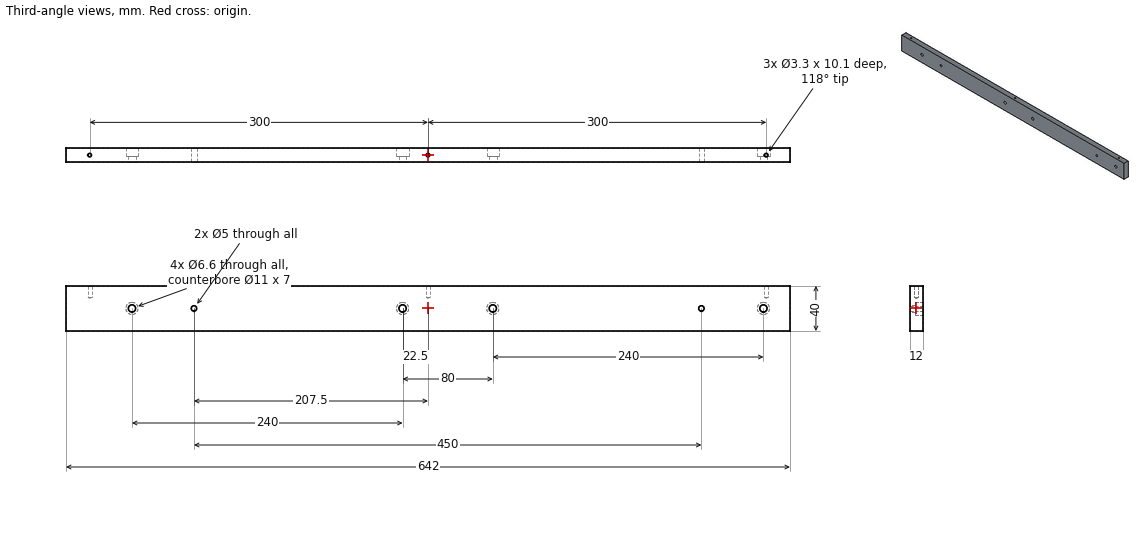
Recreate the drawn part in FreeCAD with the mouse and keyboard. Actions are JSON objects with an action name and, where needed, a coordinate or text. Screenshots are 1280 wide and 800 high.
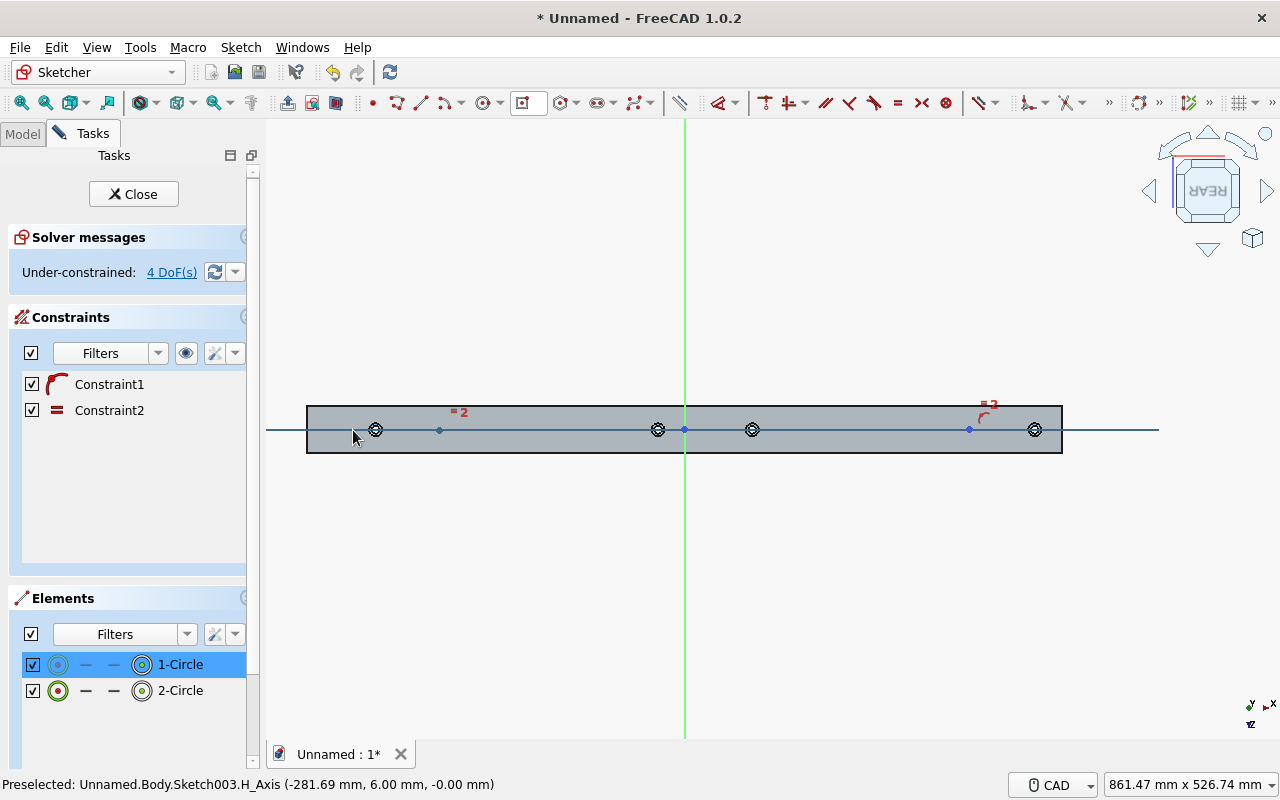
{"action": "left_click", "coordinate": [766, 104]}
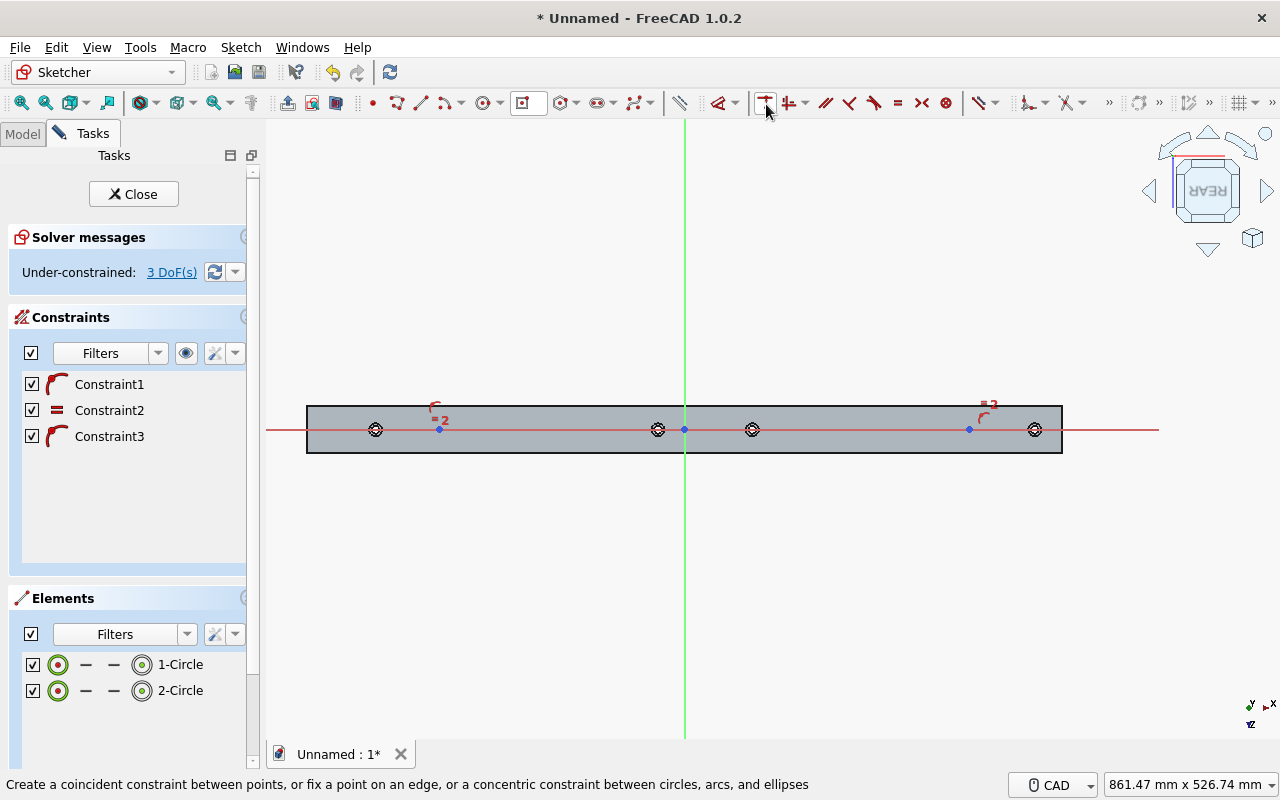
{"action": "left_click", "coordinate": [718, 104]}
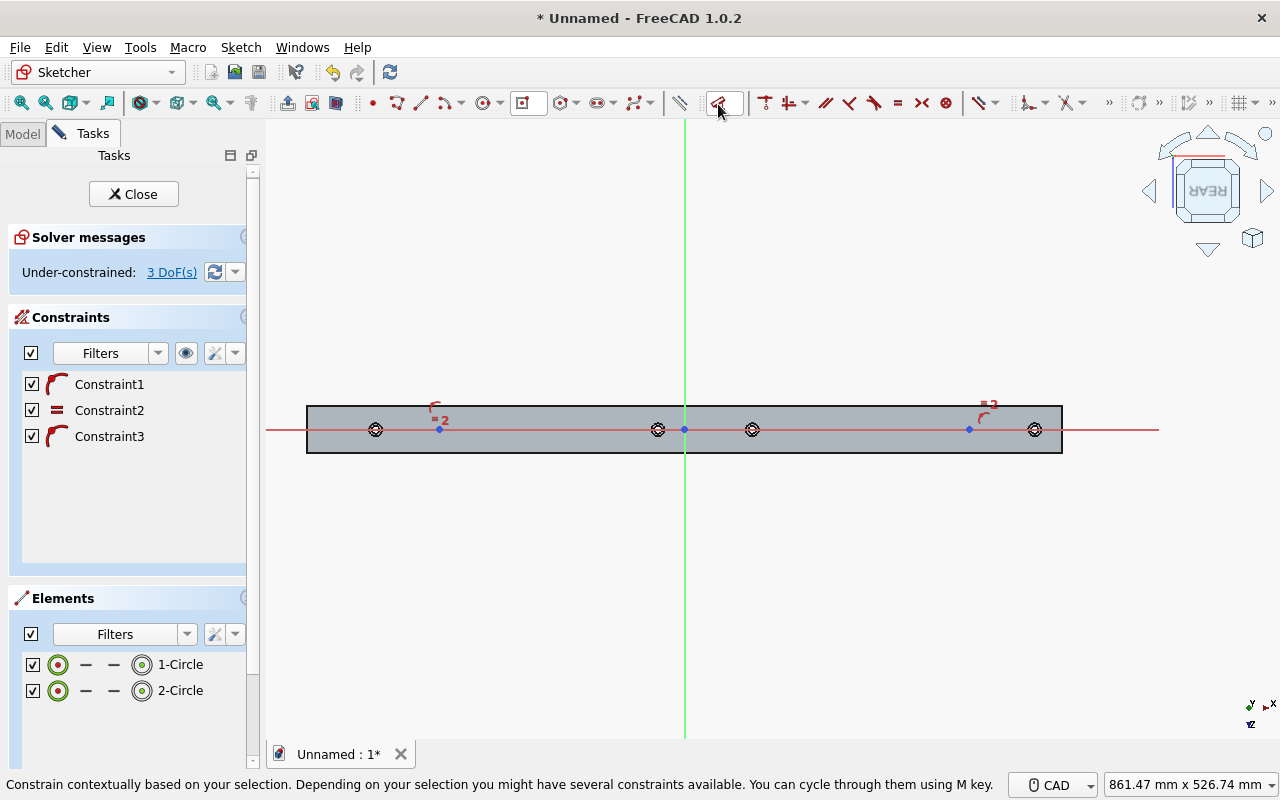
{"action": "scroll", "coordinate": [438, 430], "scroll_direction": "up", "scroll_amount": 11}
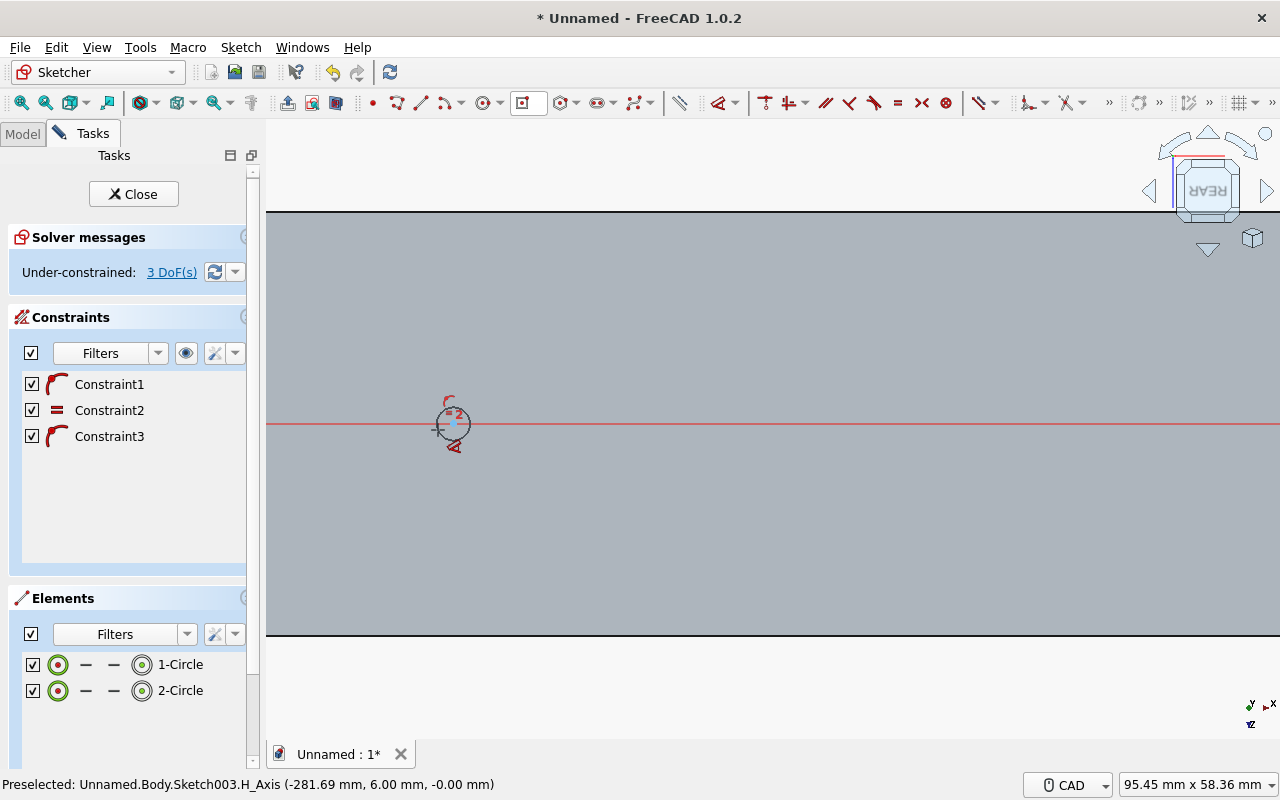
{"action": "left_click", "coordinate": [437, 424]}
{"action": "left_click", "coordinate": [411, 401]}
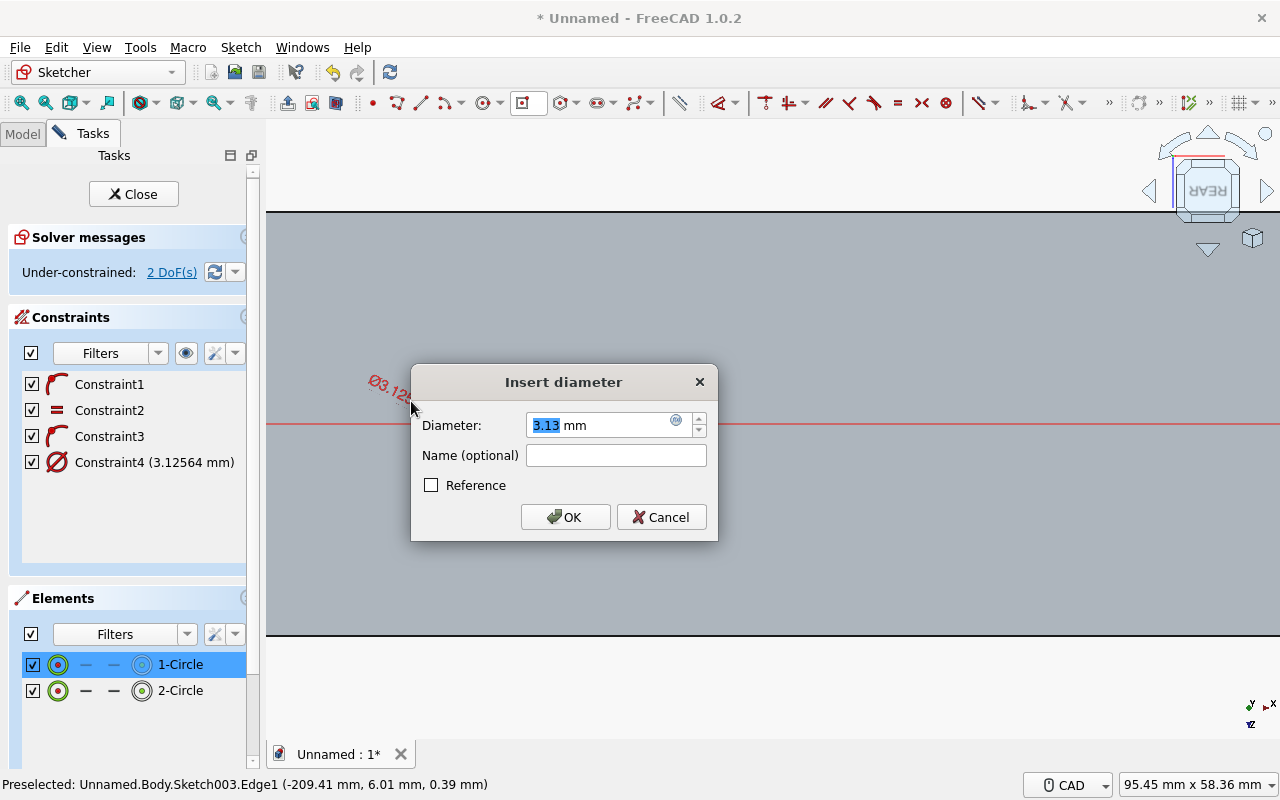
{"action": "type", "text": "5"}
{"action": "key", "text": "Return"}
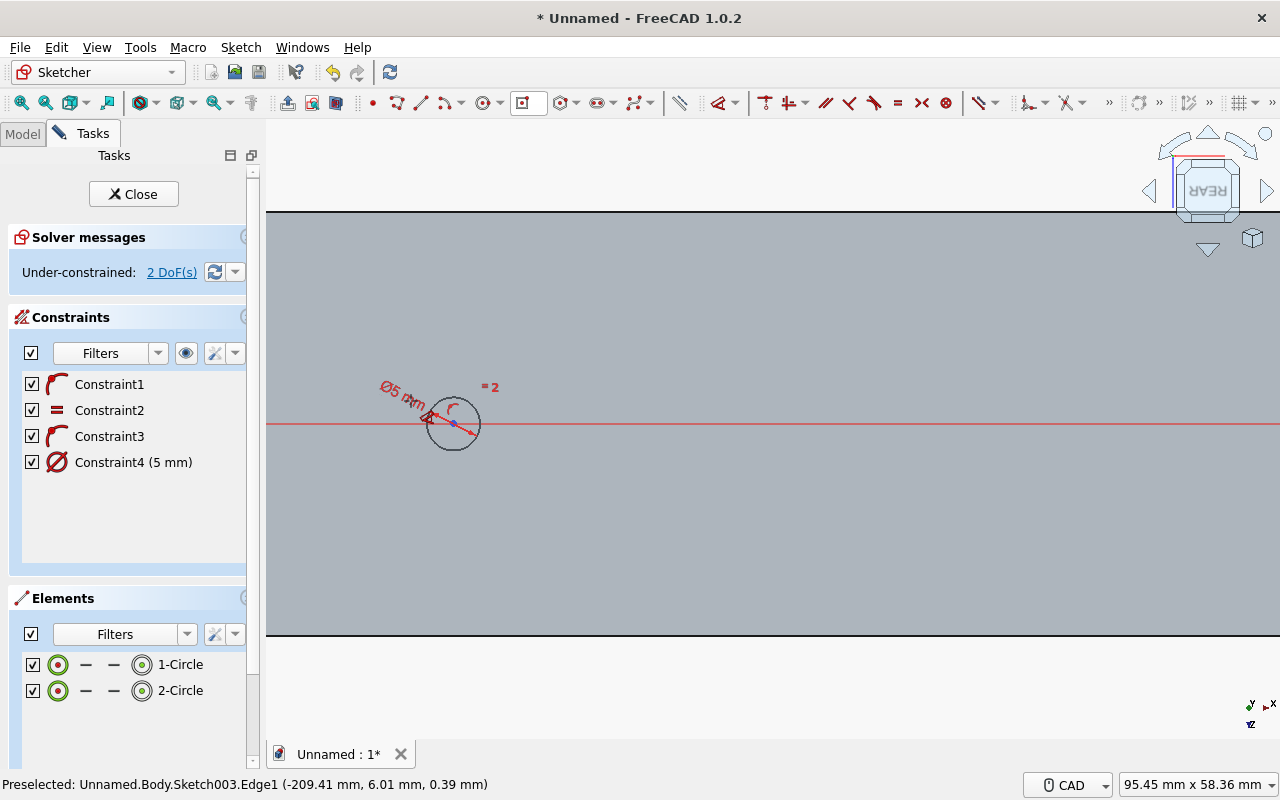
{"action": "scroll", "coordinate": [437, 430], "scroll_direction": "down", "scroll_amount": 11}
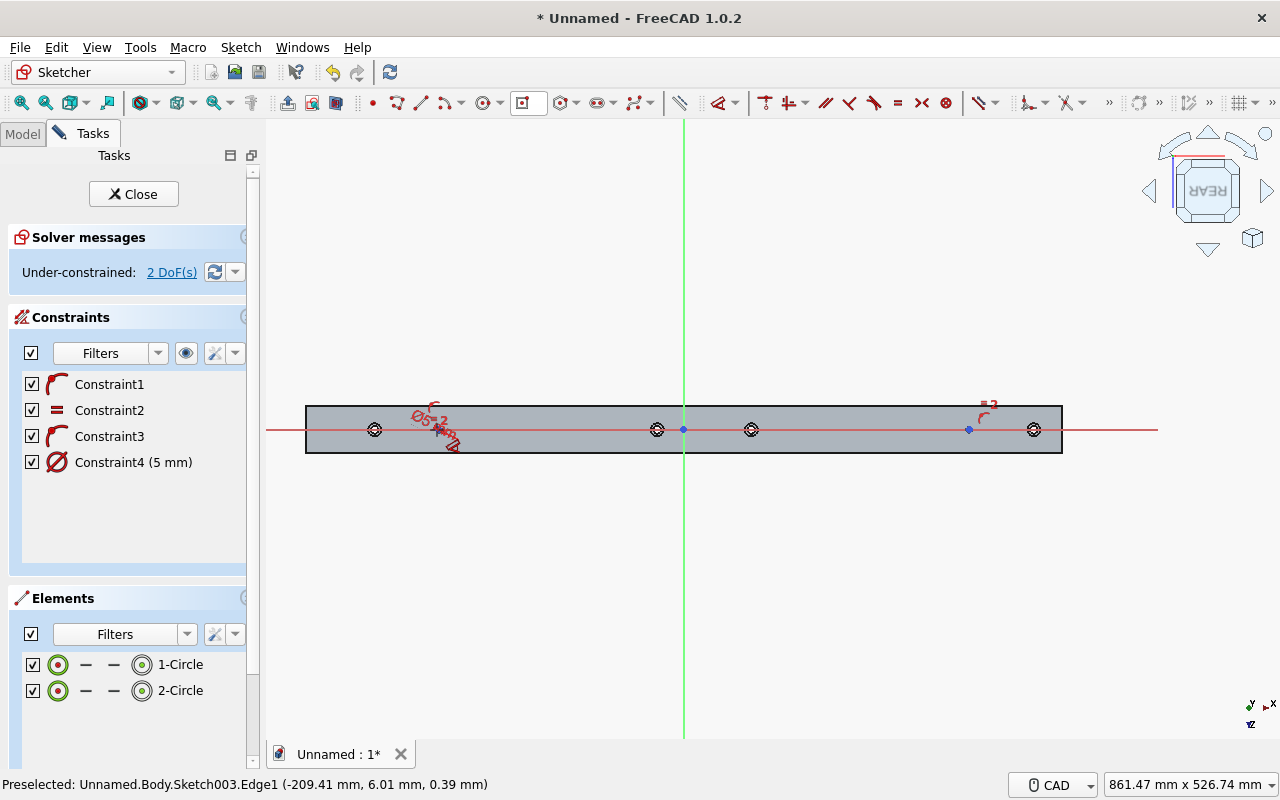
{"action": "left_click", "coordinate": [439, 430]}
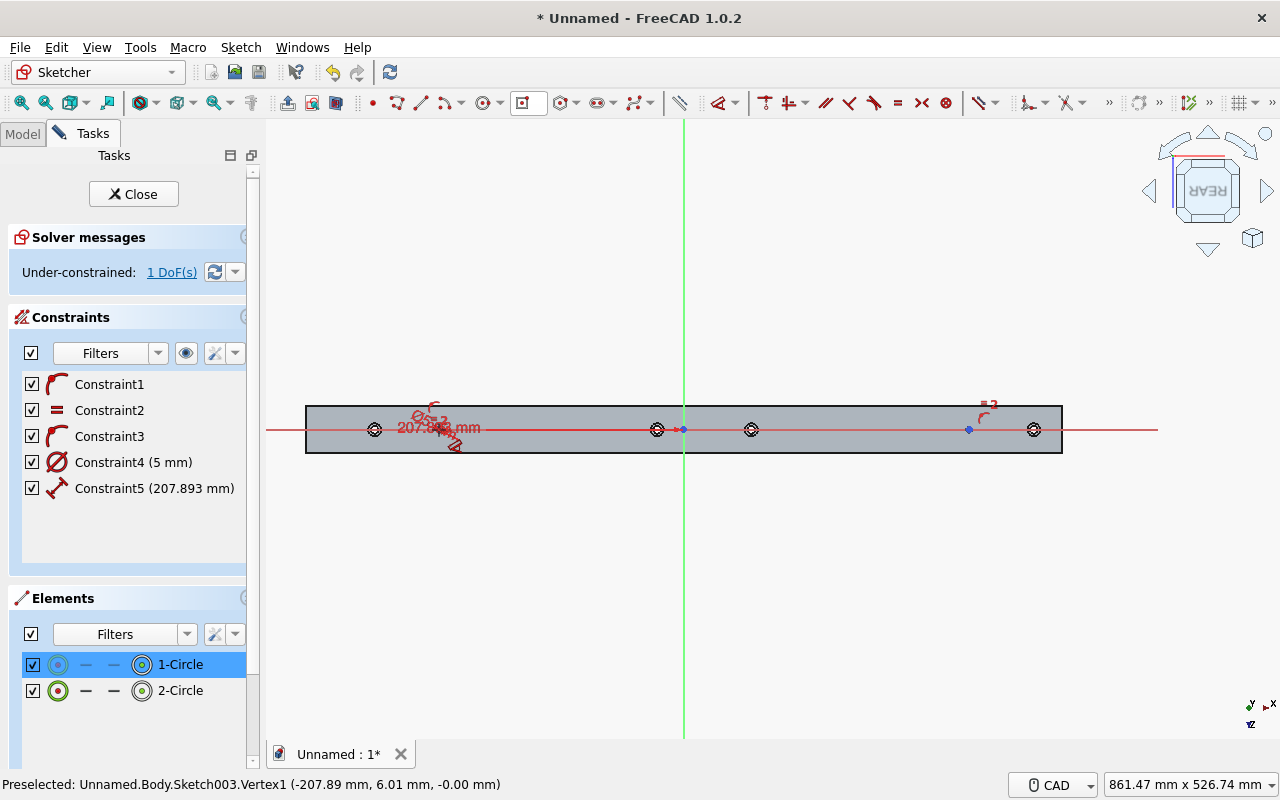
{"action": "left_click", "coordinate": [969, 430]}
{"action": "left_click", "coordinate": [704, 464]}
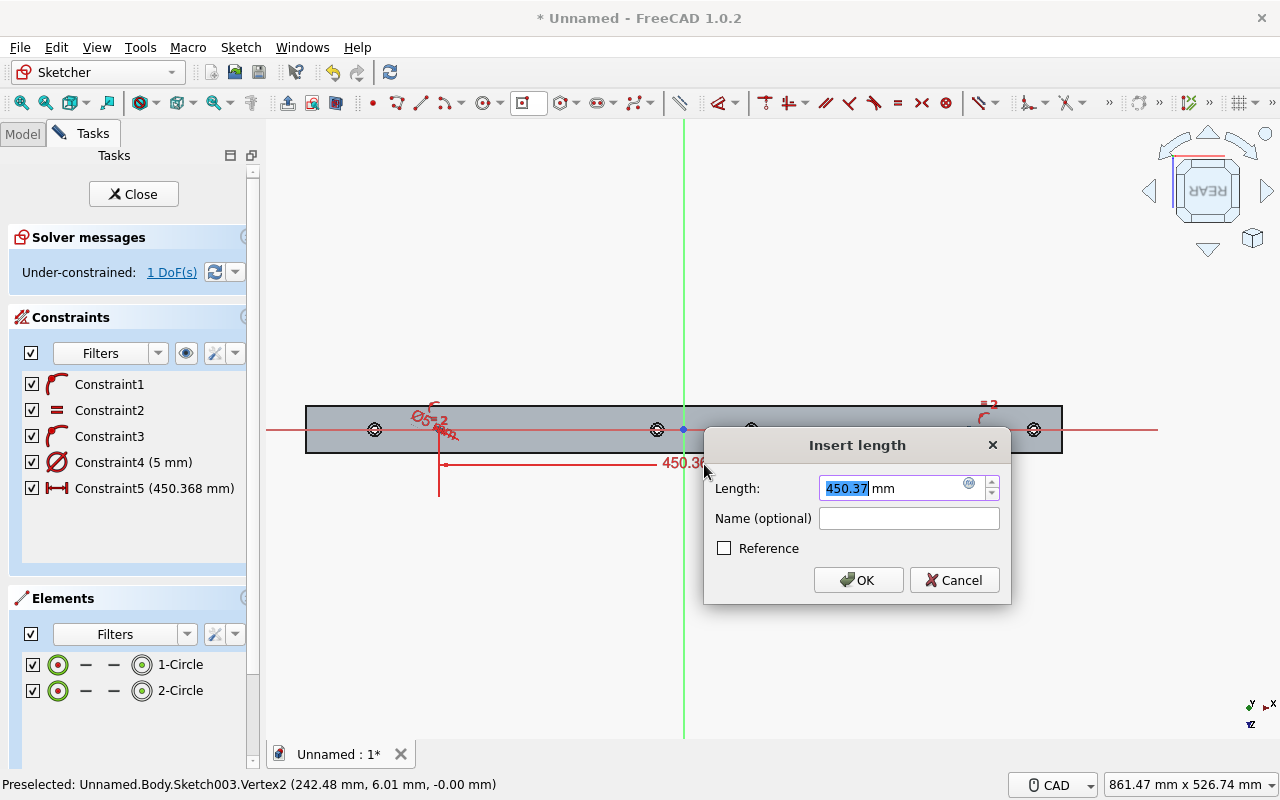
{"action": "type", "text": "450"}
{"action": "key", "text": "Return"}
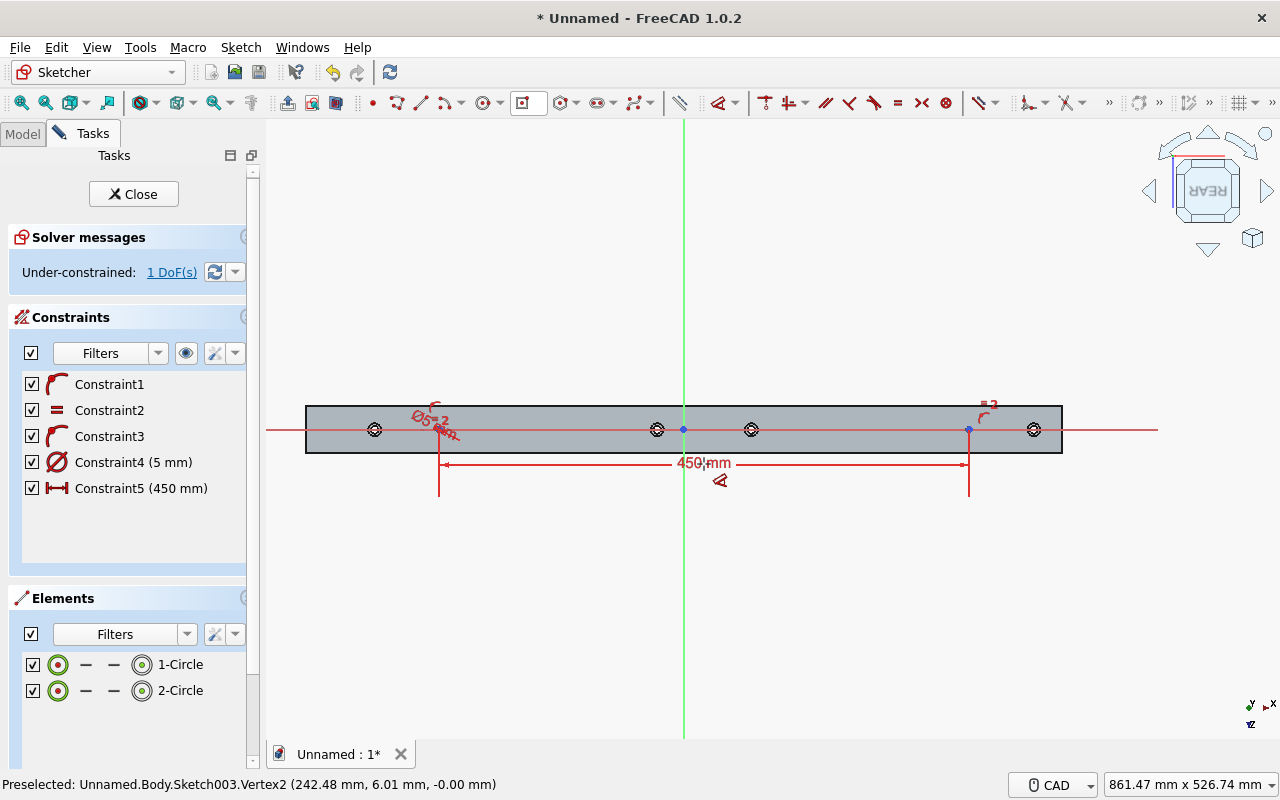
{"action": "left_click", "coordinate": [439, 430]}
{"action": "left_click", "coordinate": [562, 464]}